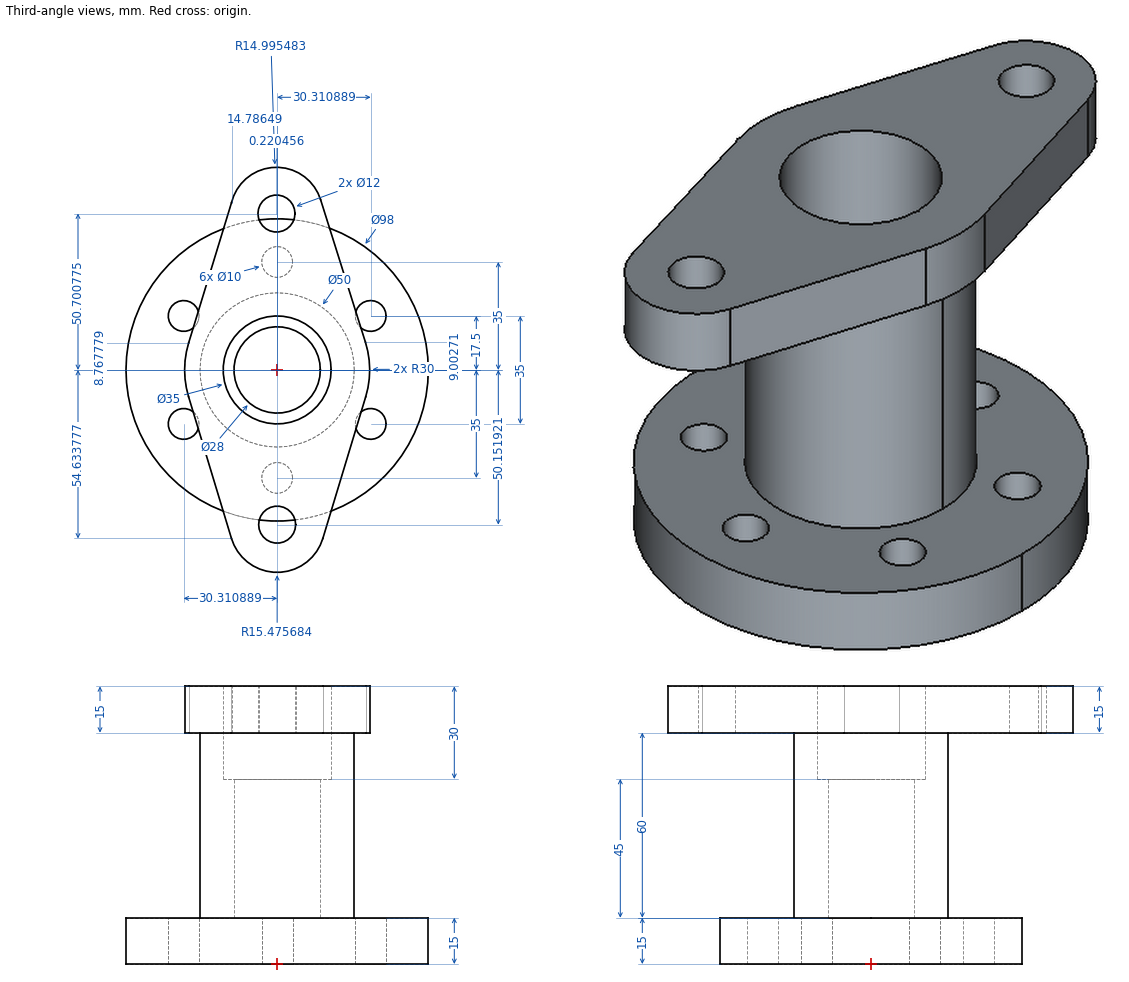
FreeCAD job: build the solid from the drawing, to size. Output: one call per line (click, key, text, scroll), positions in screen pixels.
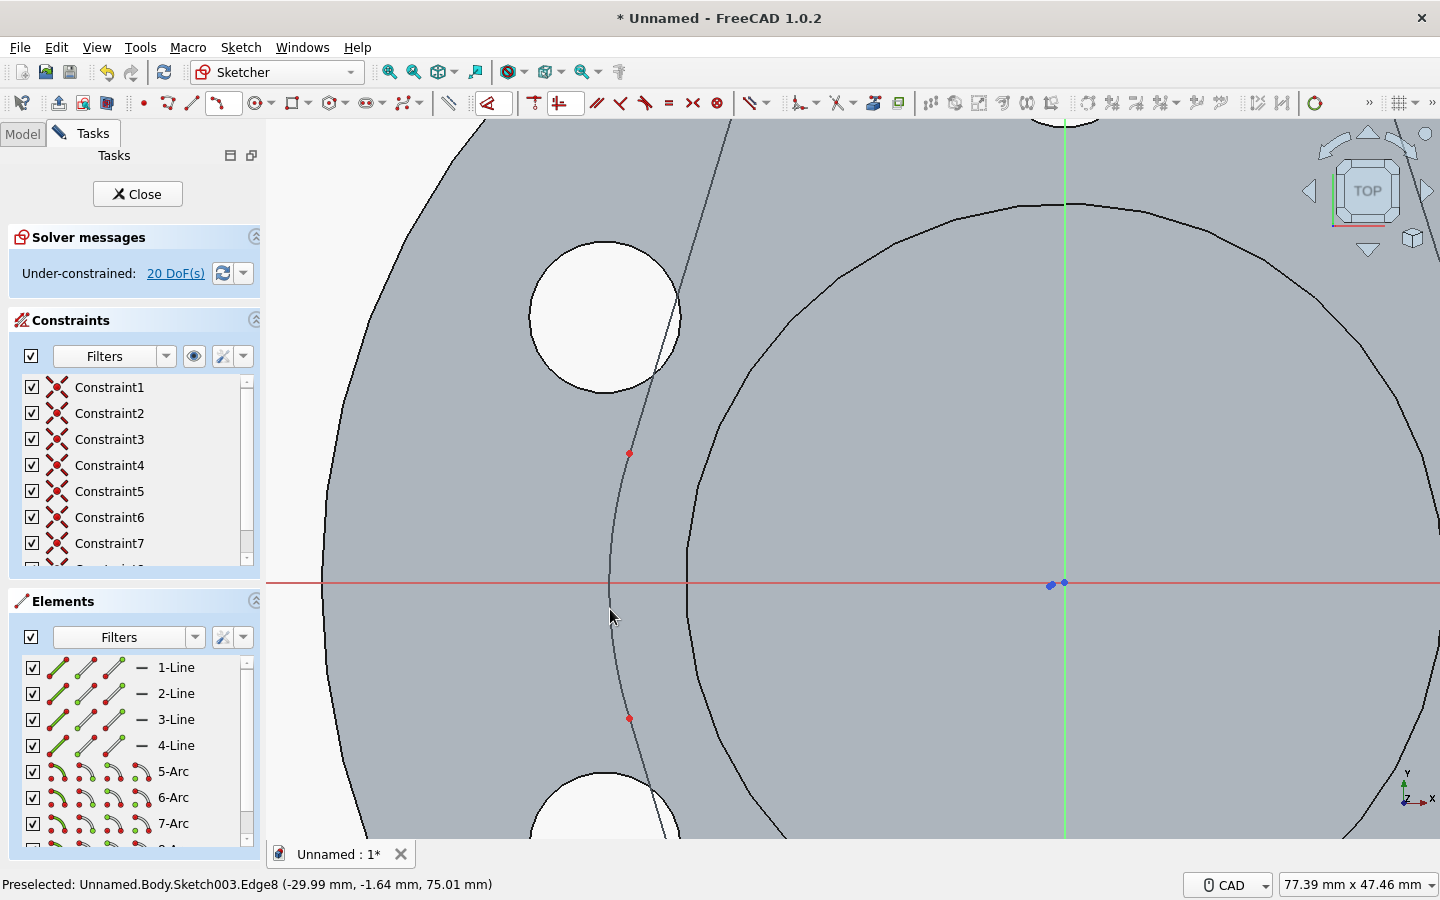
scroll(693, 445, down, 7)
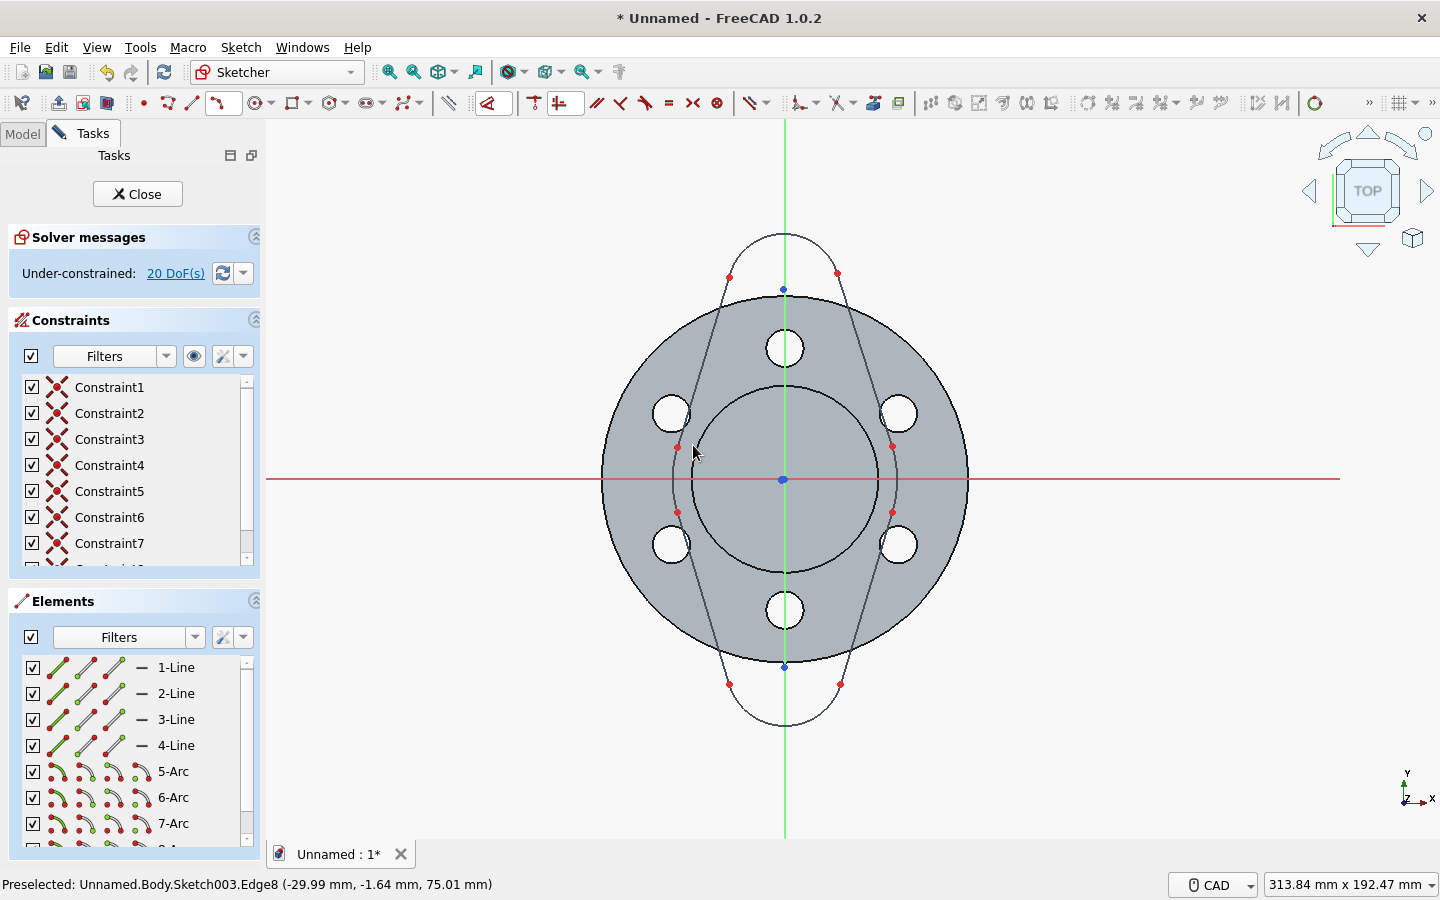
click(693, 564)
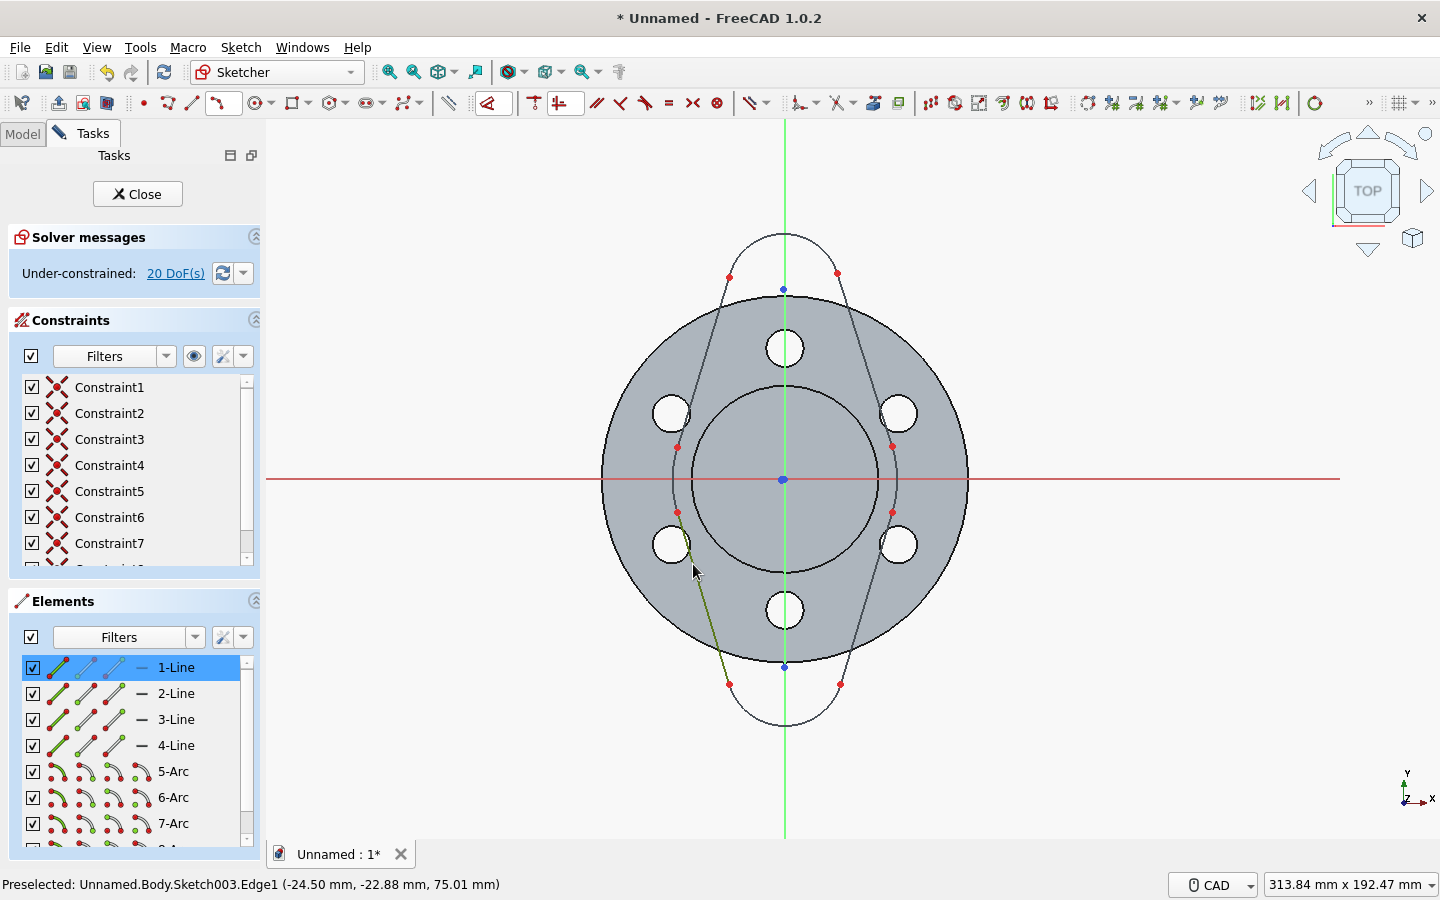
click(757, 719)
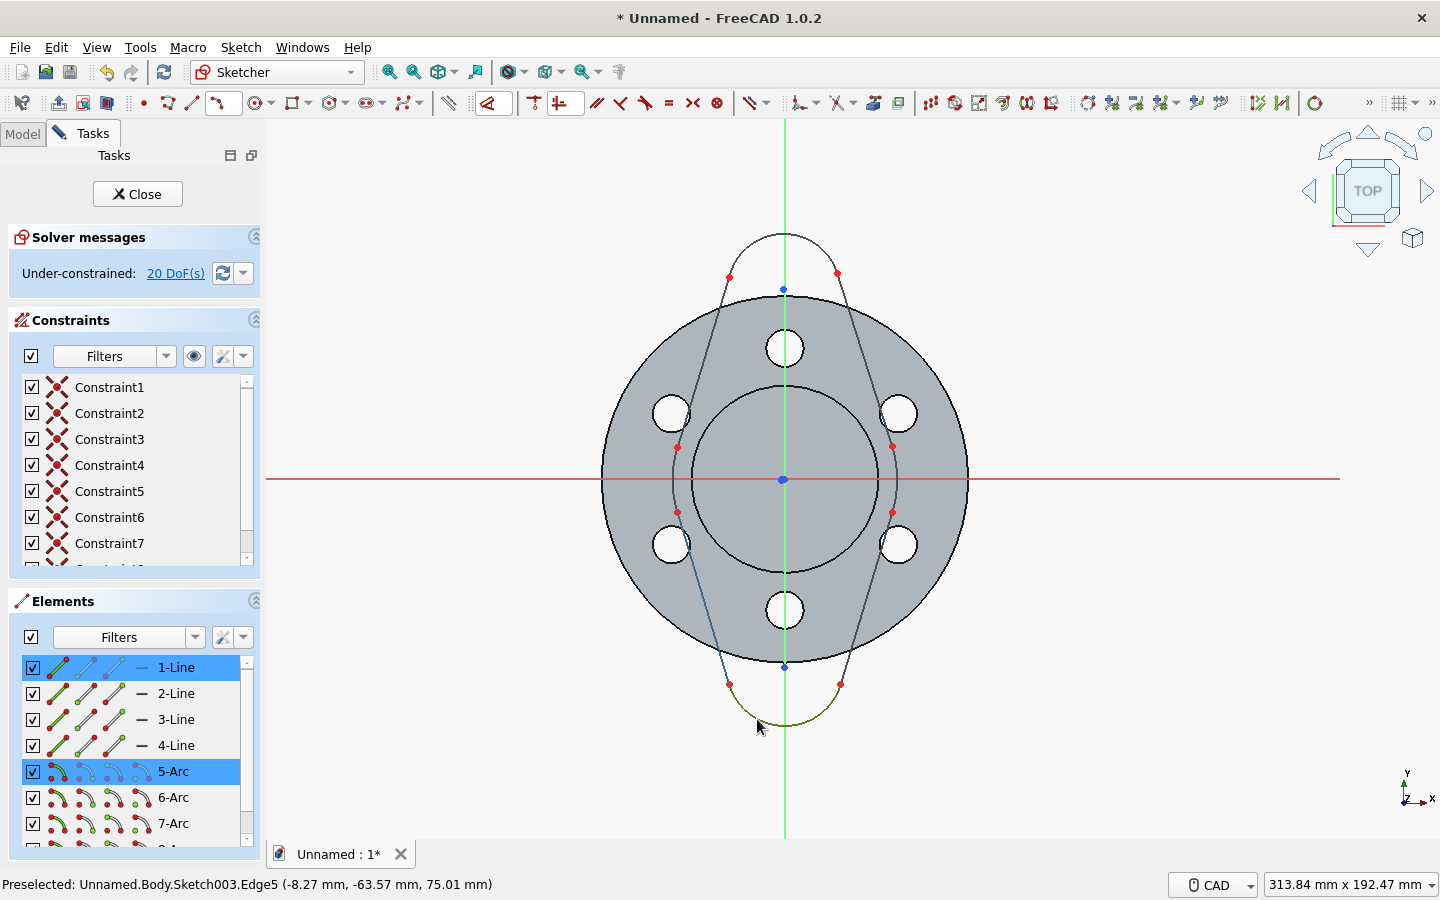
key(t)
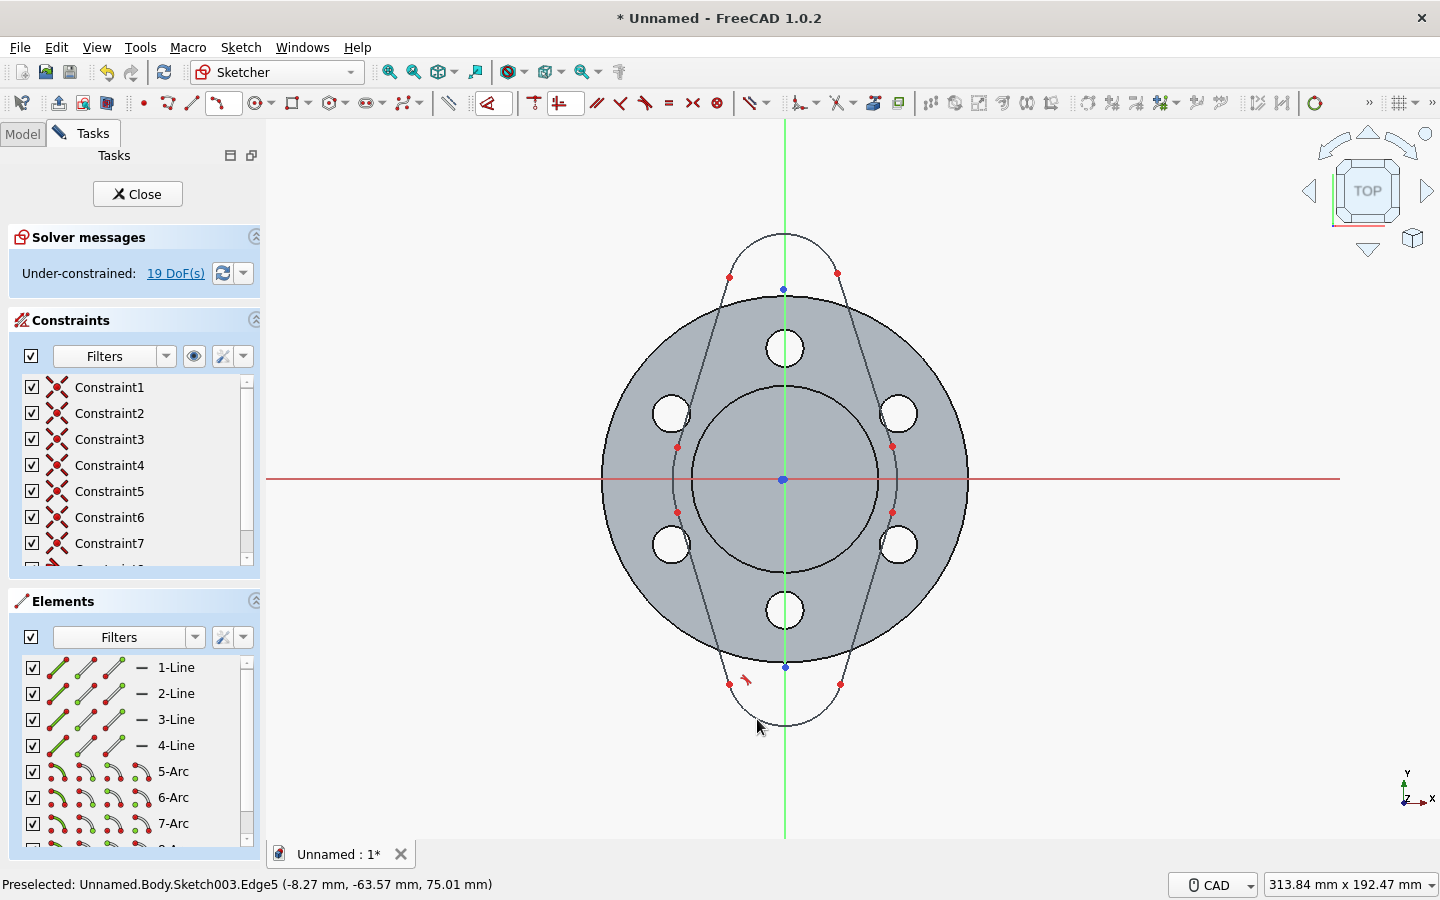
click(693, 564)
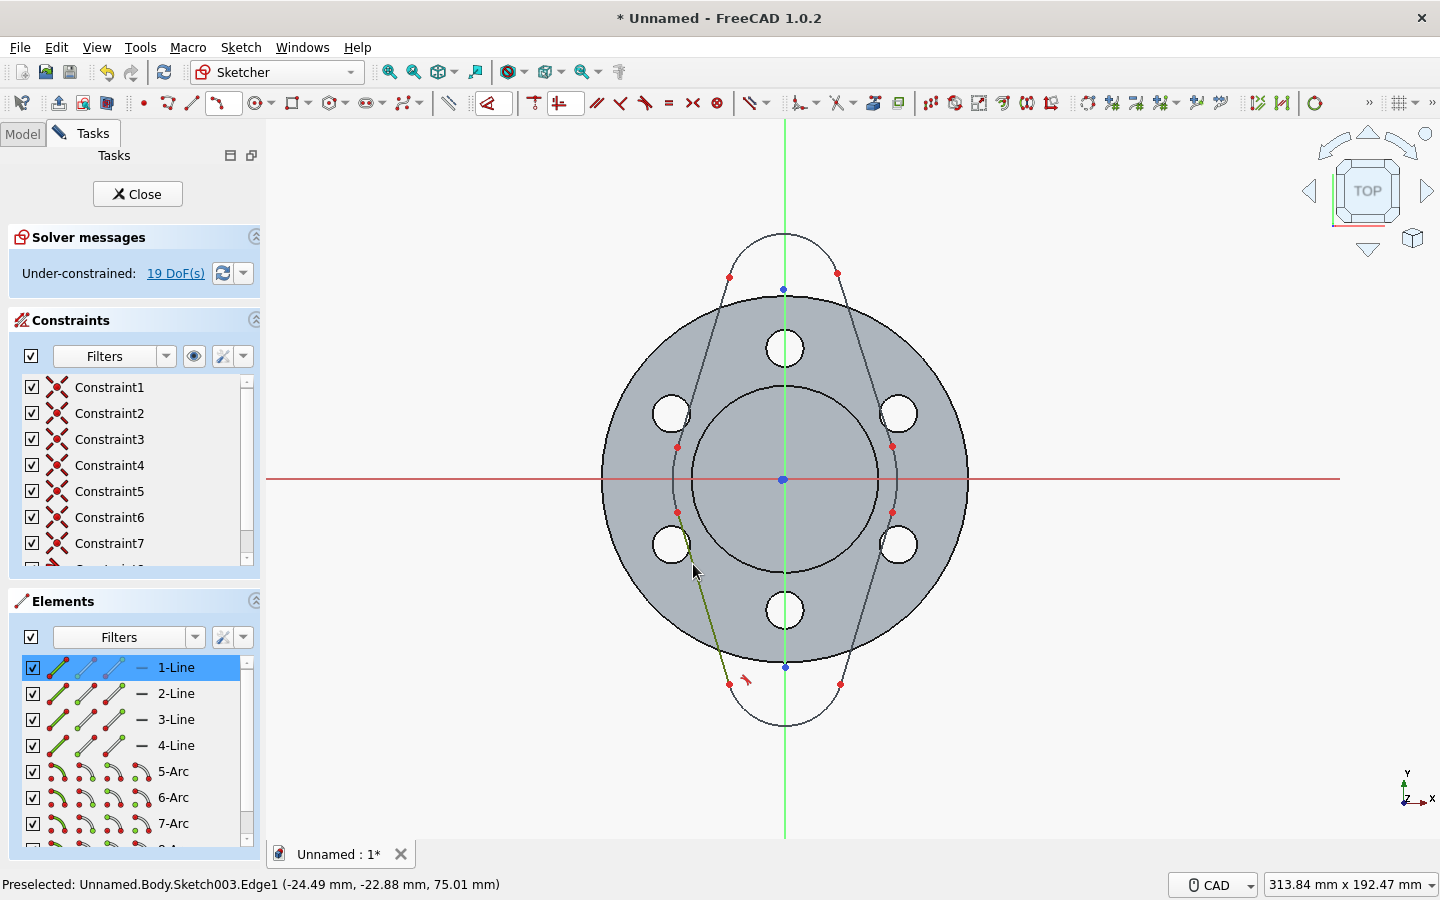
click(673, 467)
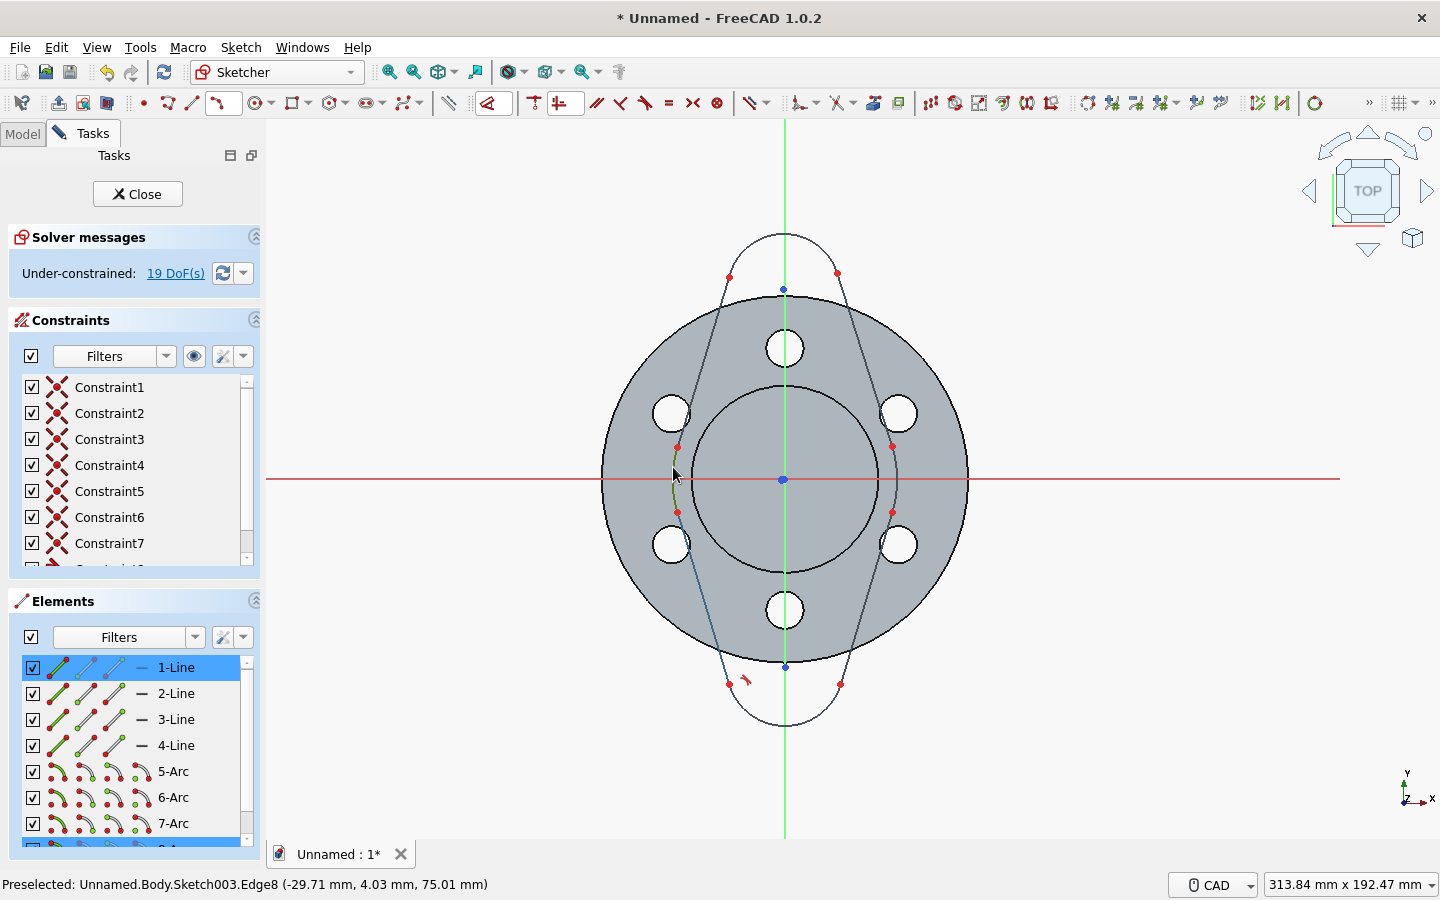
key(t)